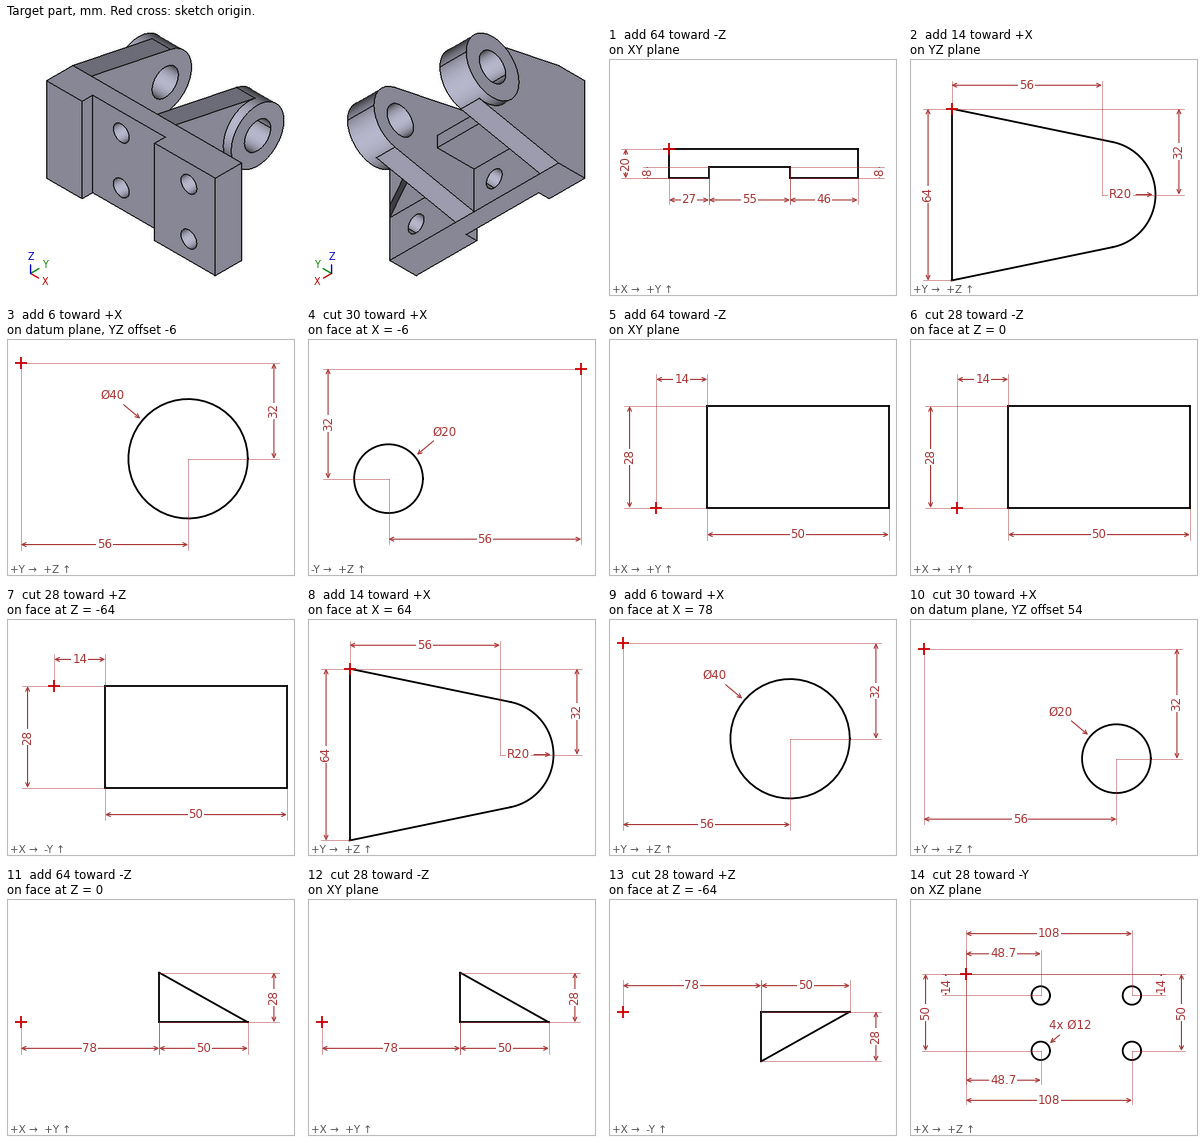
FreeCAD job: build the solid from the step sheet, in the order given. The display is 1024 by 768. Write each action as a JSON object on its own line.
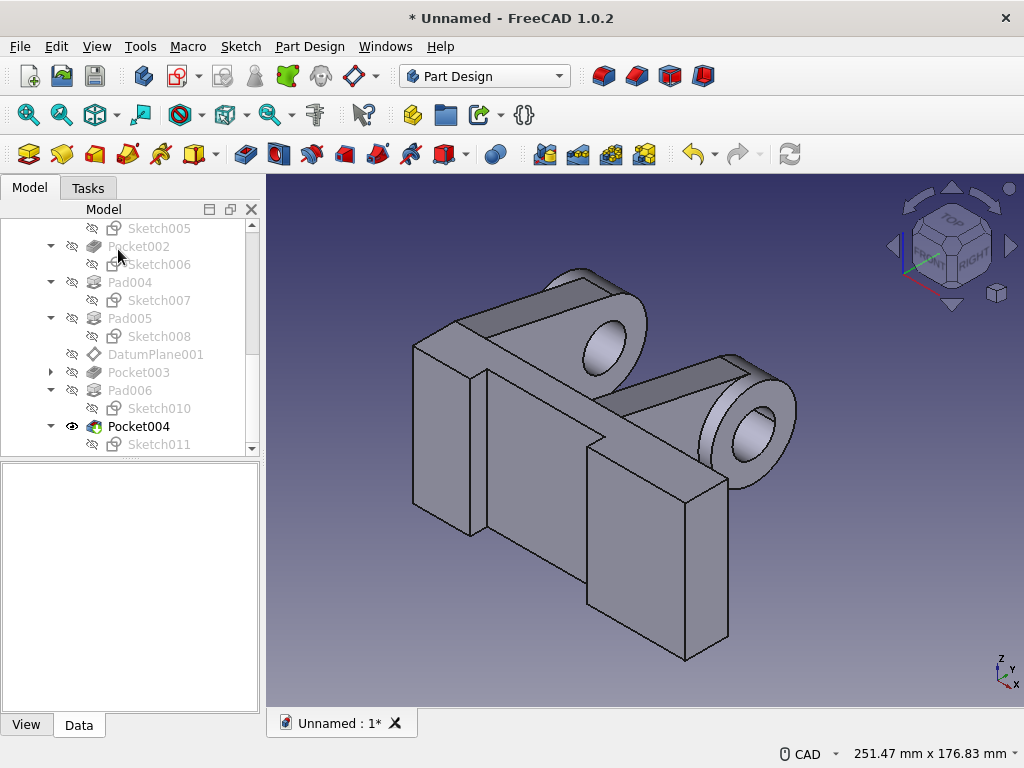
{"action": "key", "text": "5"}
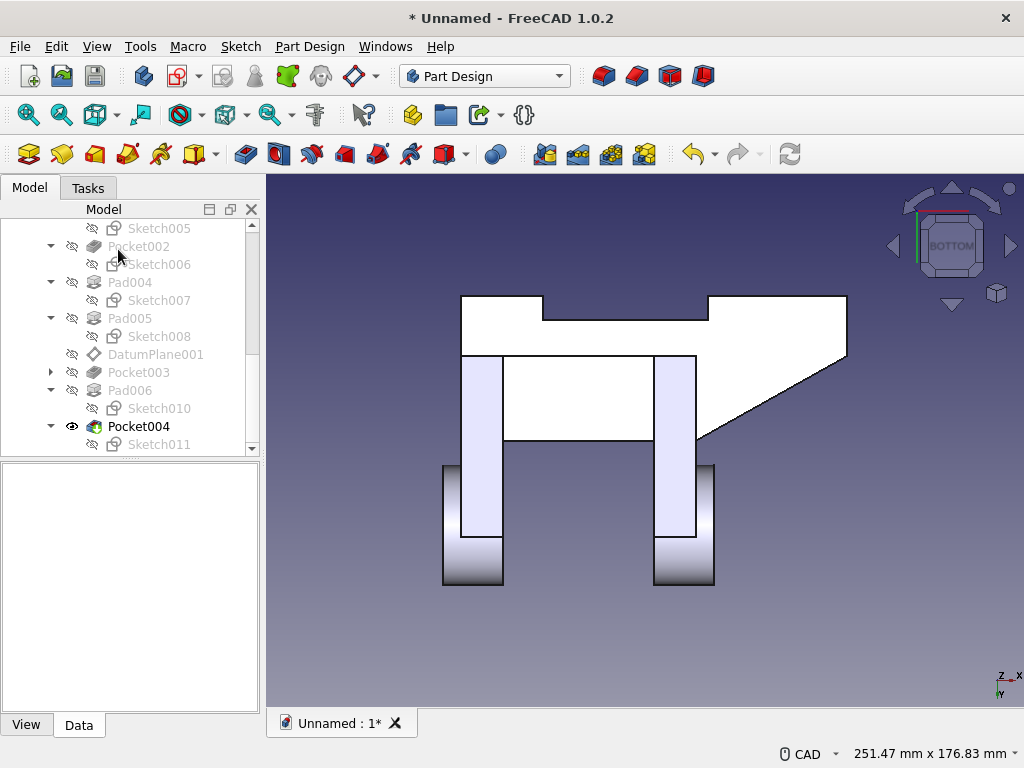
{"action": "left_click", "coordinate": [764, 346]}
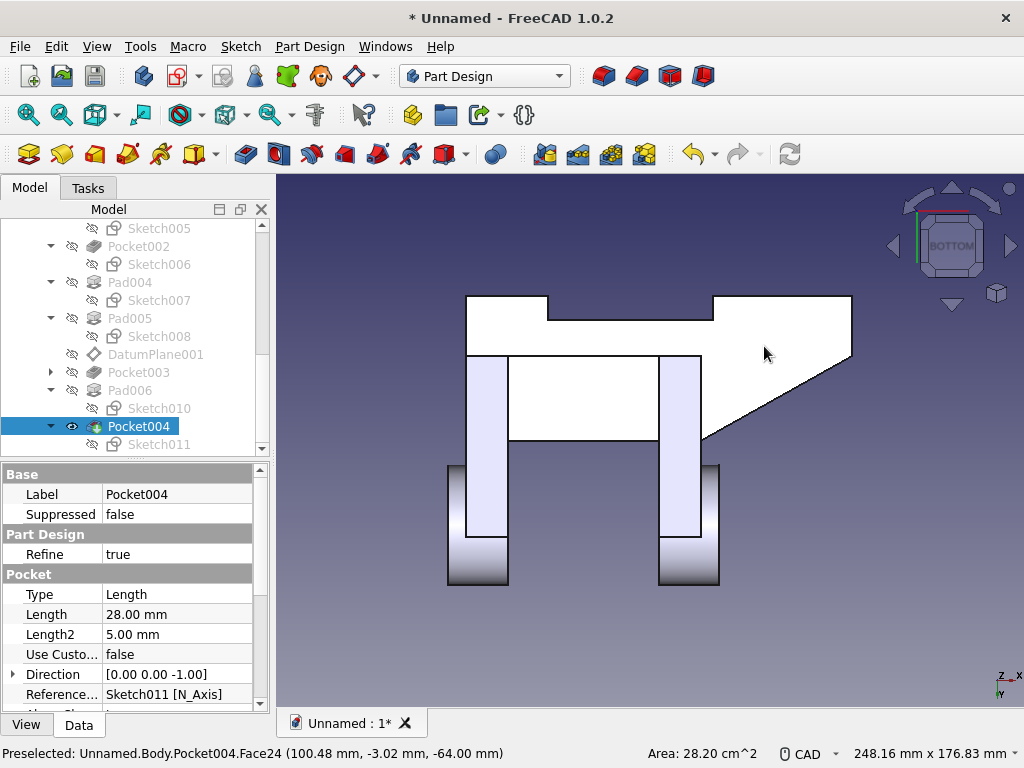
{"action": "left_click", "coordinate": [176, 76]}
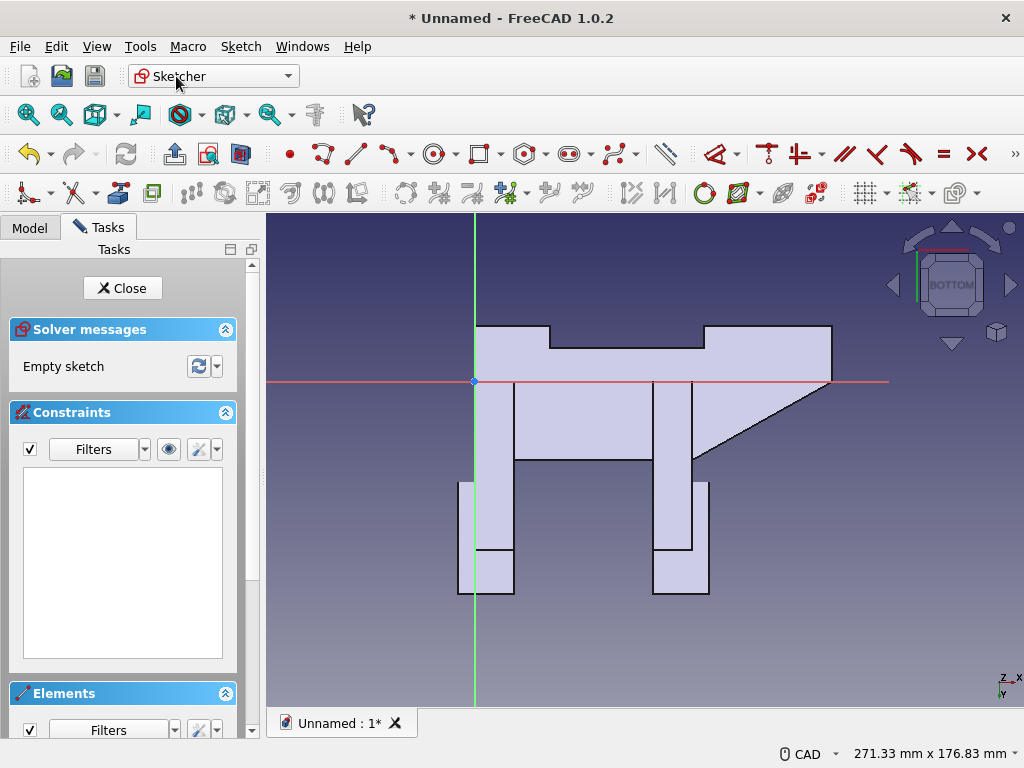
{"action": "scroll", "coordinate": [859, 398], "scroll_direction": "up", "scroll_amount": 5}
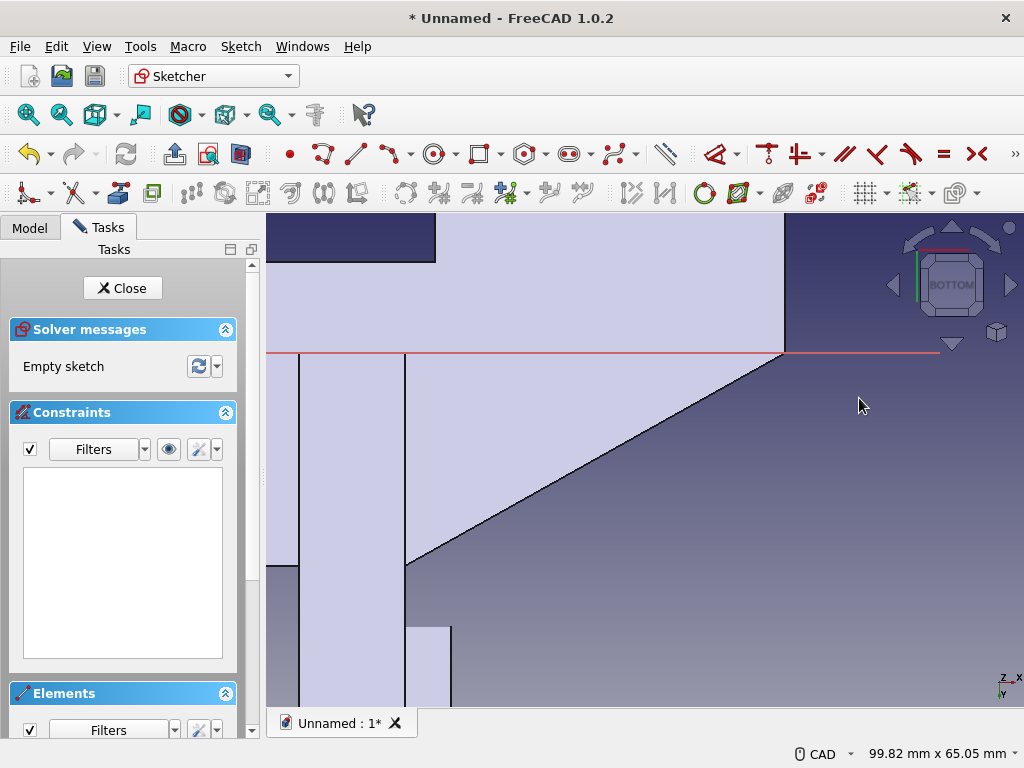
{"action": "left_click", "coordinate": [323, 154]}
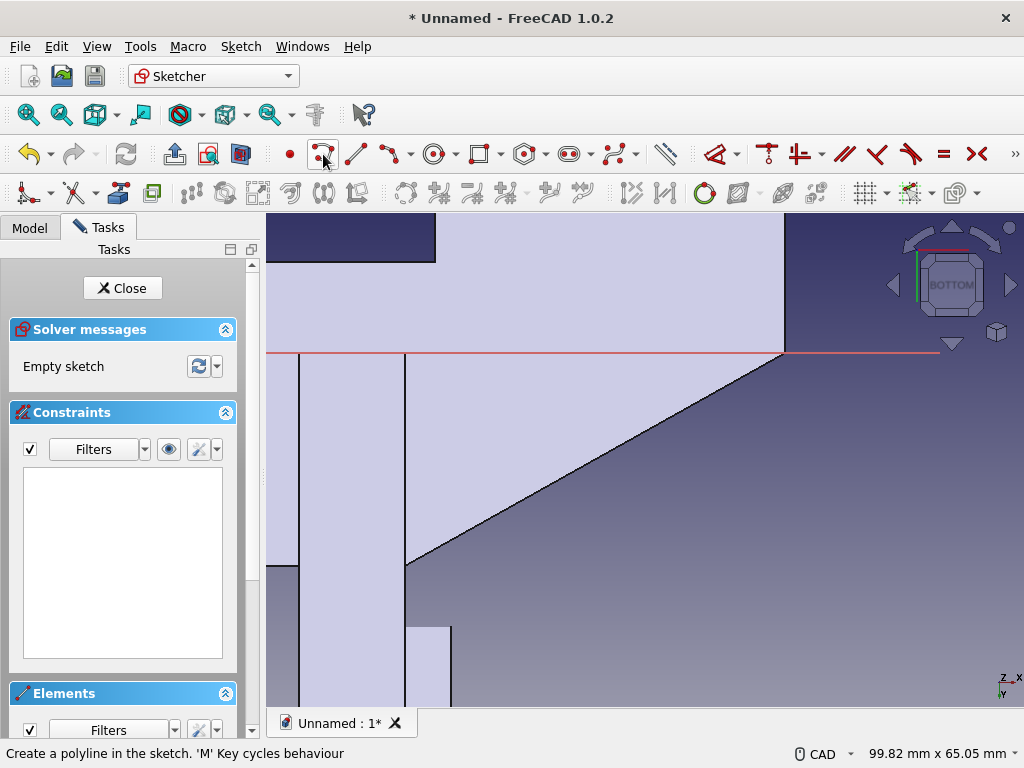
{"action": "left_click", "coordinate": [405, 353]}
{"action": "left_click", "coordinate": [405, 566]}
{"action": "left_click", "coordinate": [785, 362]}
{"action": "left_click", "coordinate": [405, 353]}
{"action": "key", "text": "Escape"}
{"action": "key", "text": "Escape"}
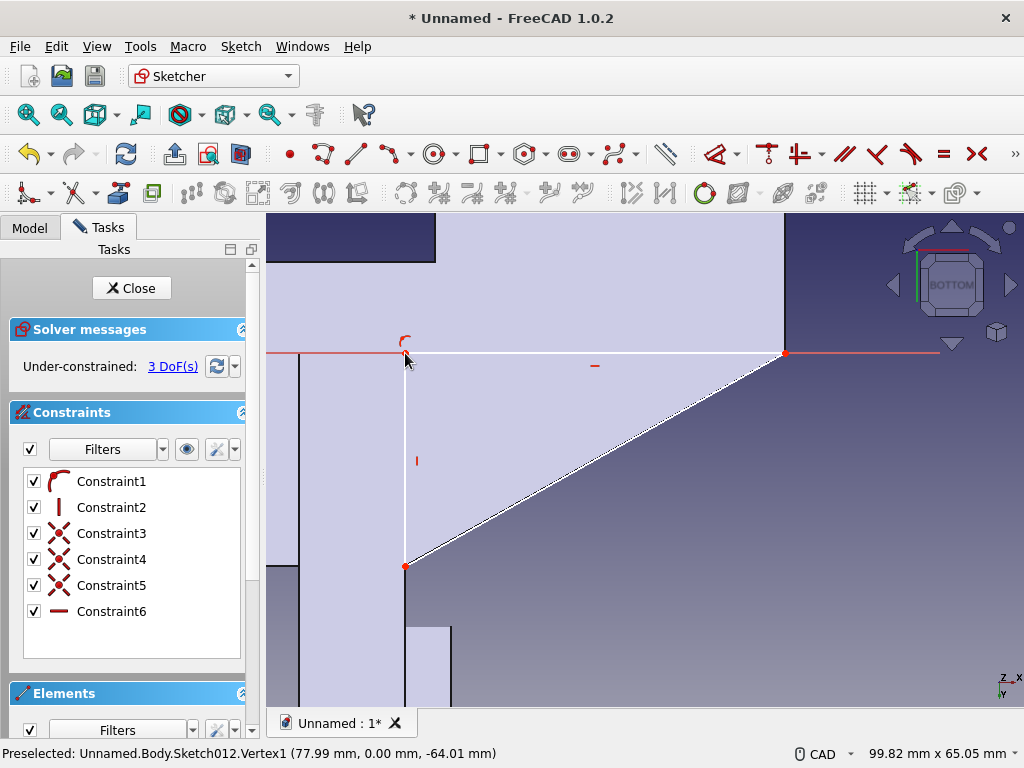
{"action": "left_click", "coordinate": [714, 154]}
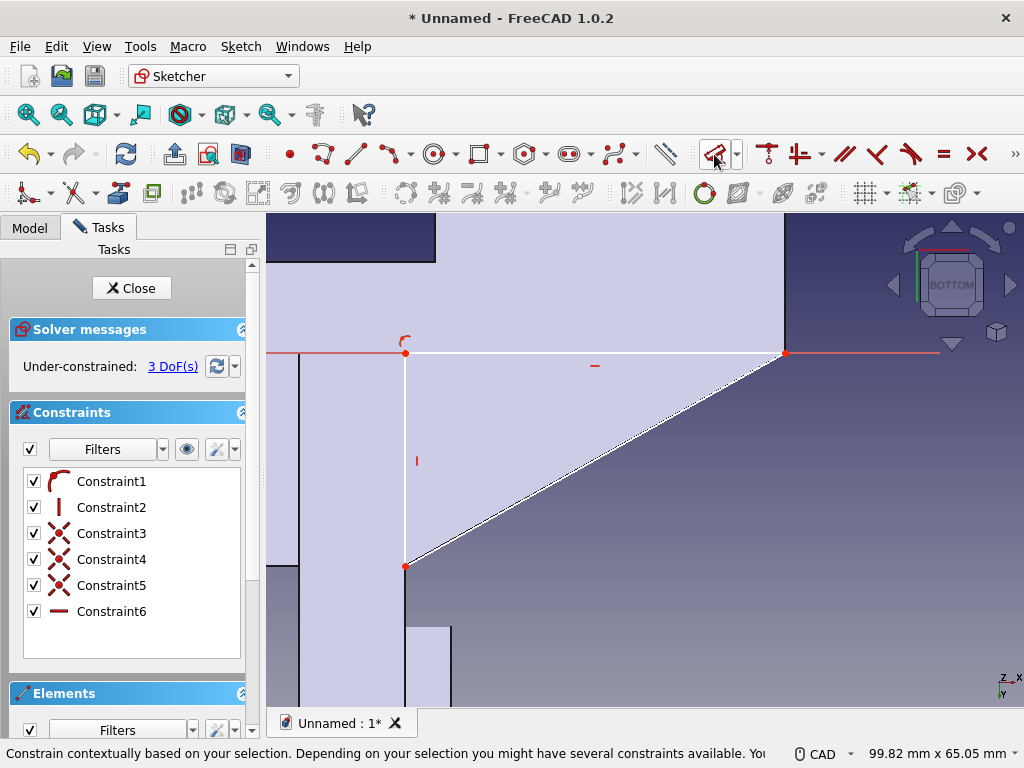
{"action": "left_click", "coordinate": [405, 417]}
{"action": "left_click", "coordinate": [371, 460]}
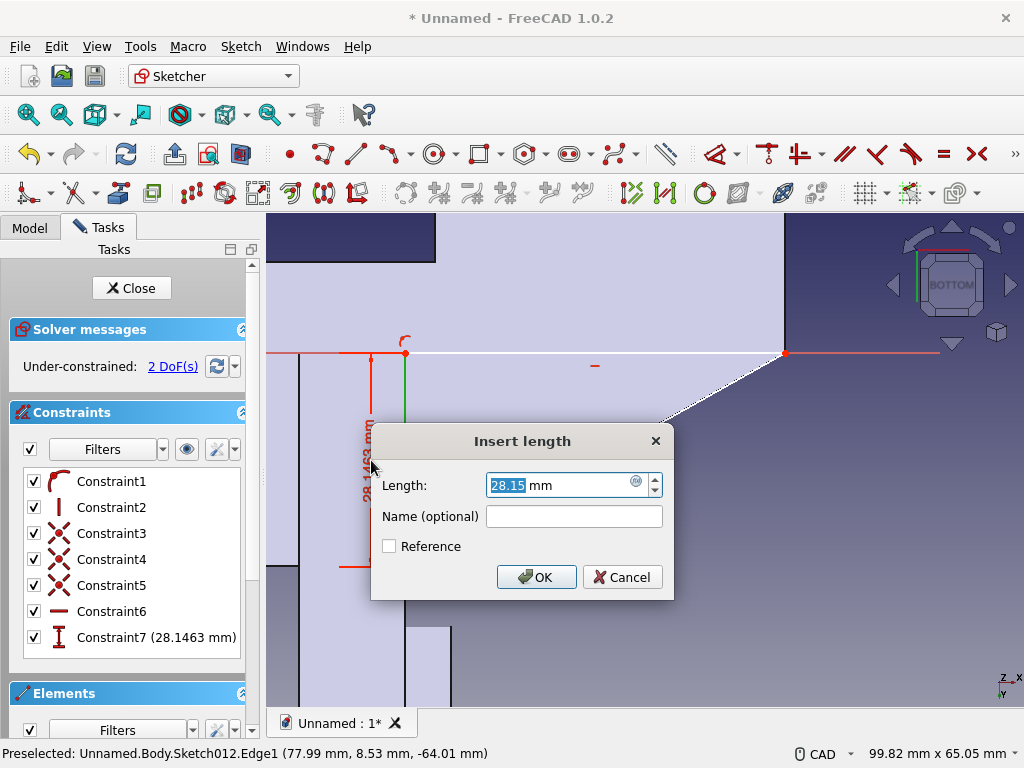
{"action": "type", "text": "28"}
{"action": "key", "text": "Return"}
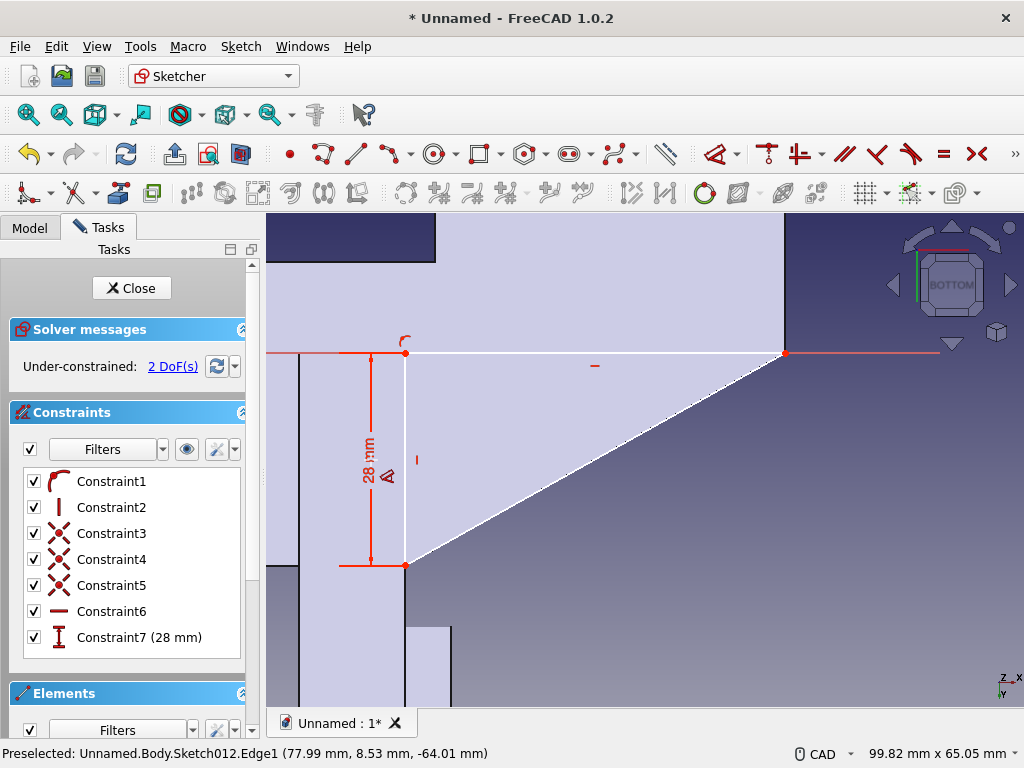
{"action": "left_click", "coordinate": [671, 353]}
{"action": "left_click", "coordinate": [595, 319]}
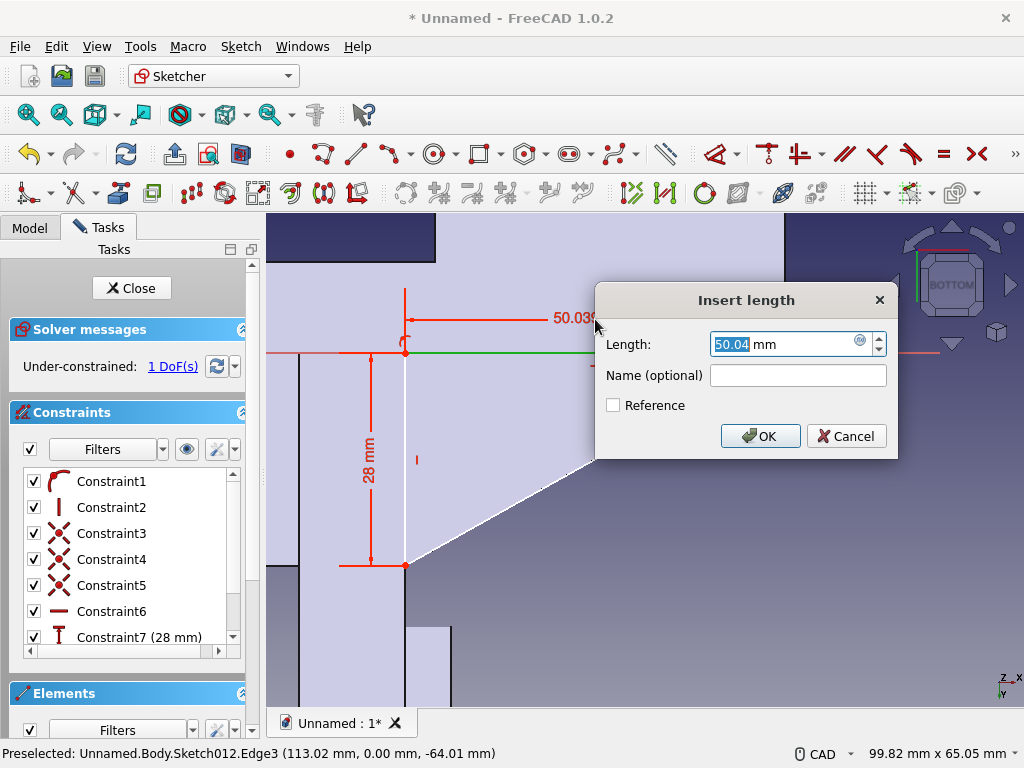
{"action": "type", "text": "50"}
{"action": "key", "text": "Return"}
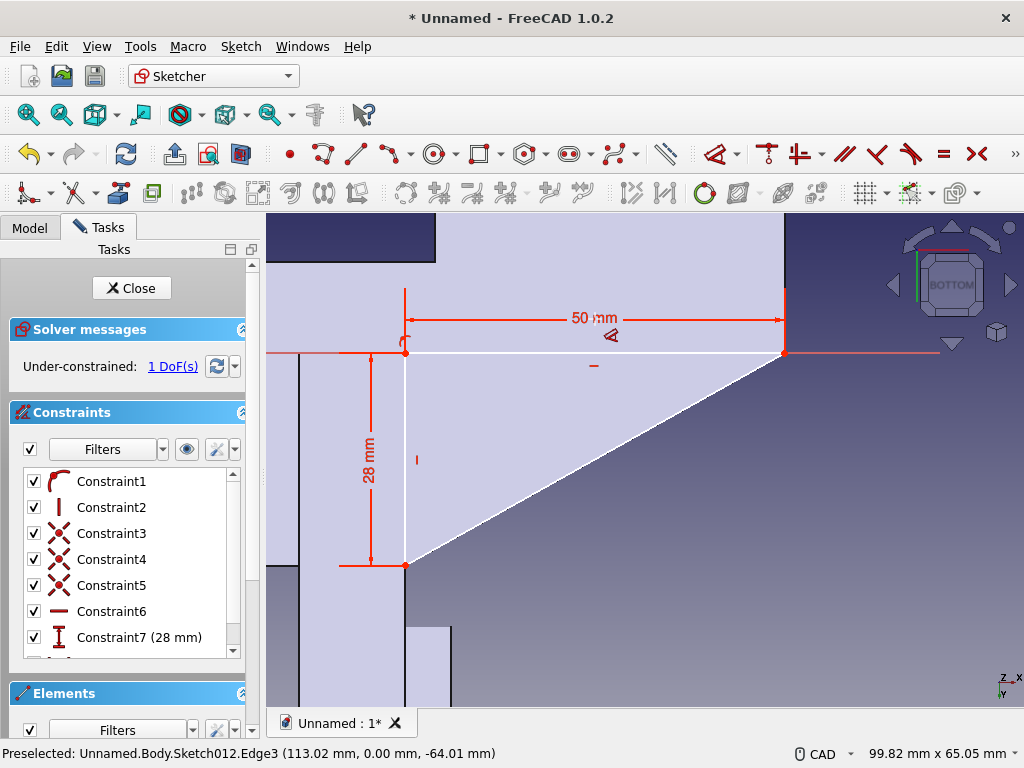
{"action": "left_click", "coordinate": [405, 353]}
{"action": "left_click", "coordinate": [350, 319]}